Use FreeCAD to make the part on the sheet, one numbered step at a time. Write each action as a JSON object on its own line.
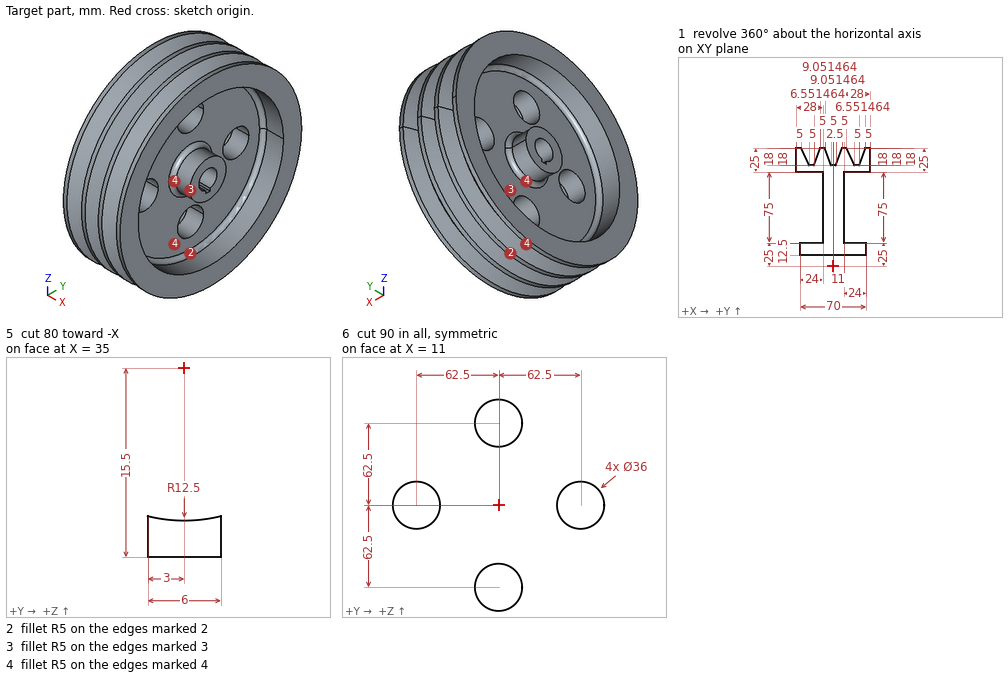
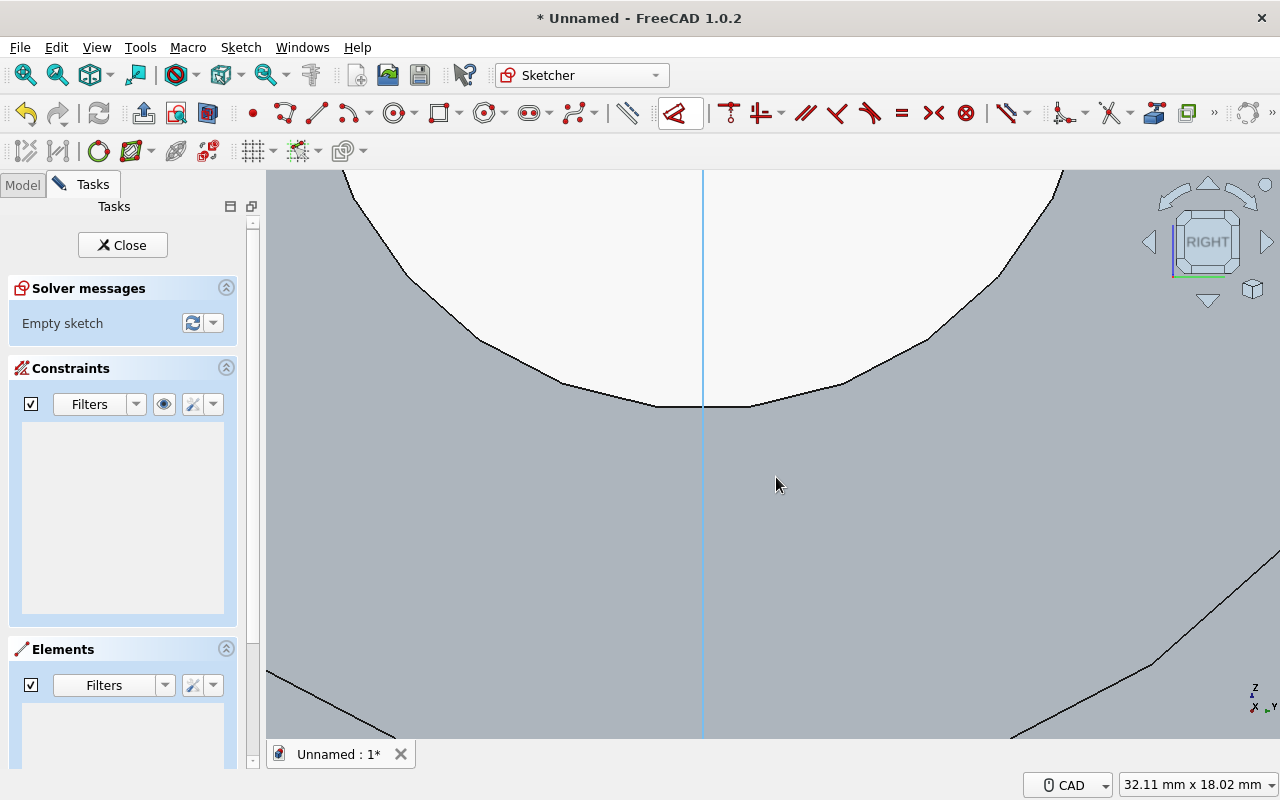
{"action": "scroll", "coordinate": [703, 450], "scroll_direction": "up", "scroll_amount": 6}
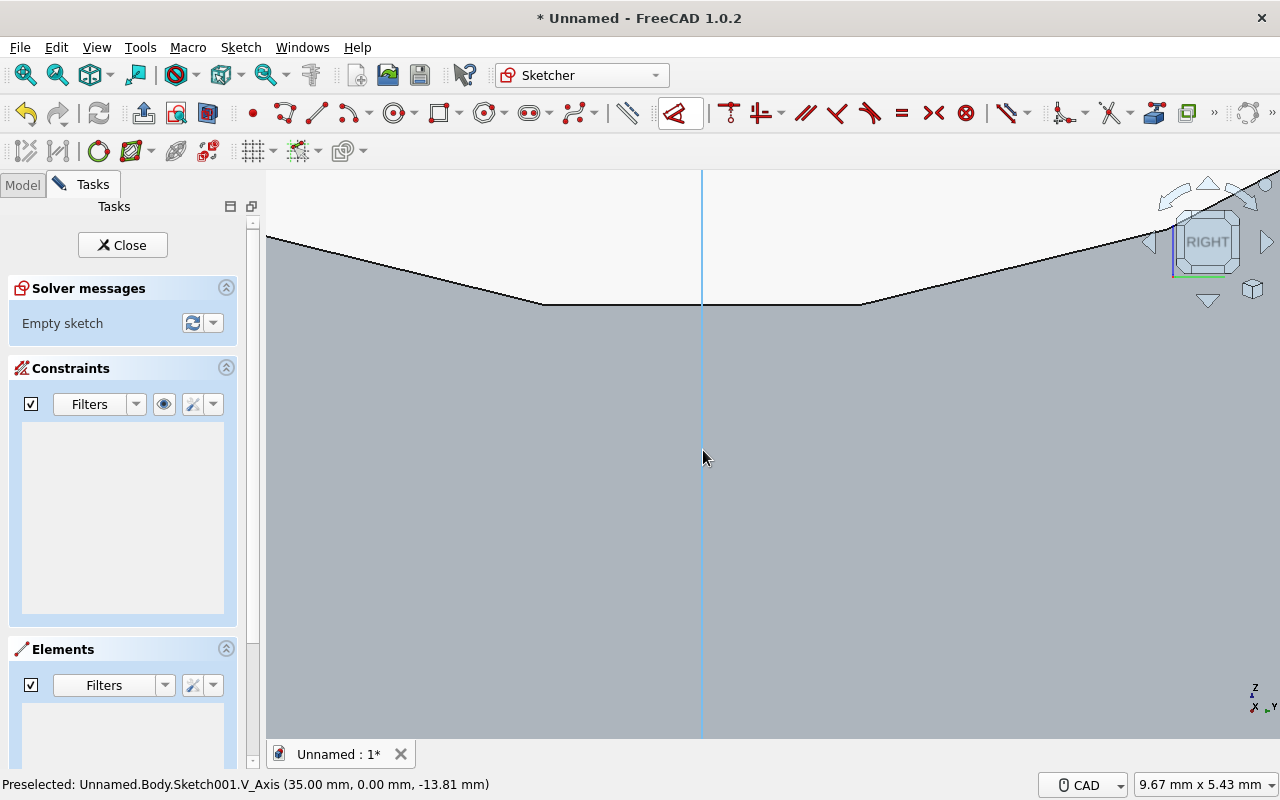
{"action": "left_click", "coordinate": [286, 114]}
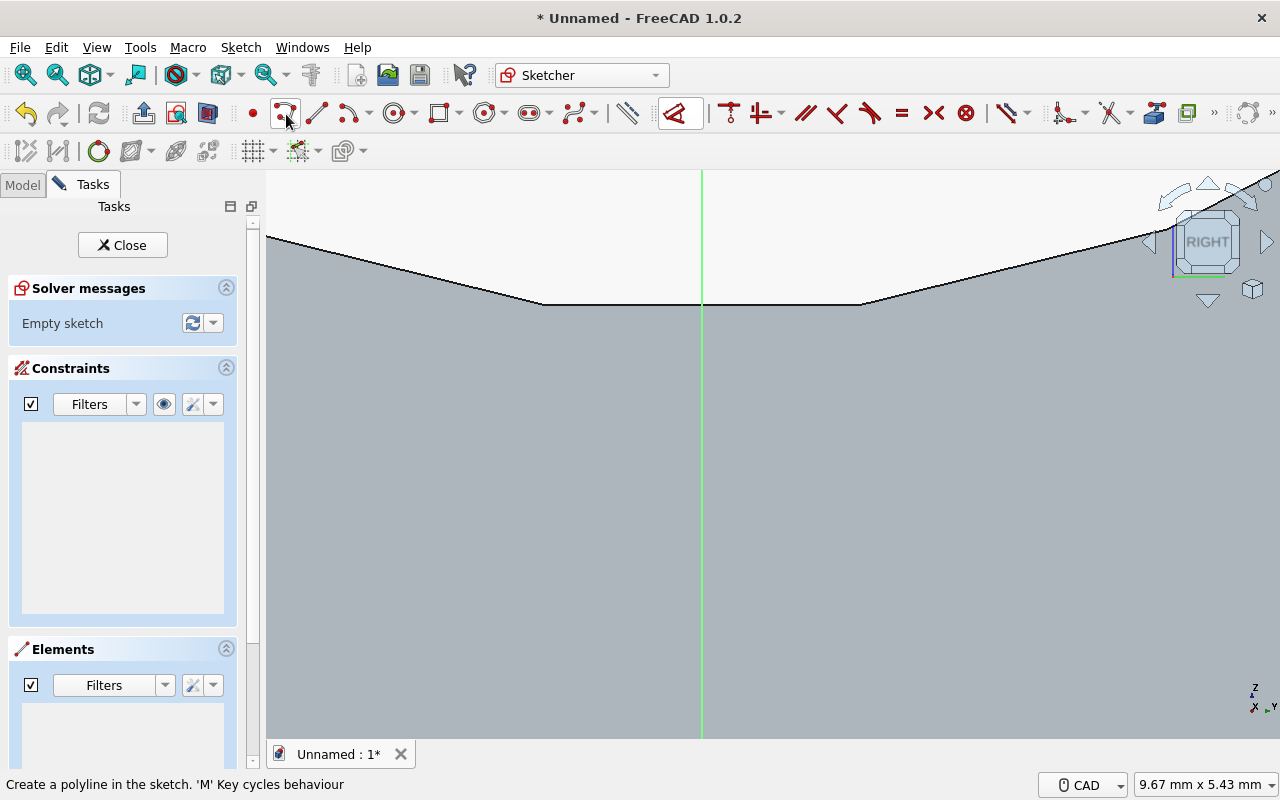
{"action": "left_click", "coordinate": [388, 276]}
{"action": "left_click", "coordinate": [388, 629]}
{"action": "left_click", "coordinate": [1017, 629]}
{"action": "left_click", "coordinate": [1017, 276]}
{"action": "right_click", "coordinate": [1017, 276]}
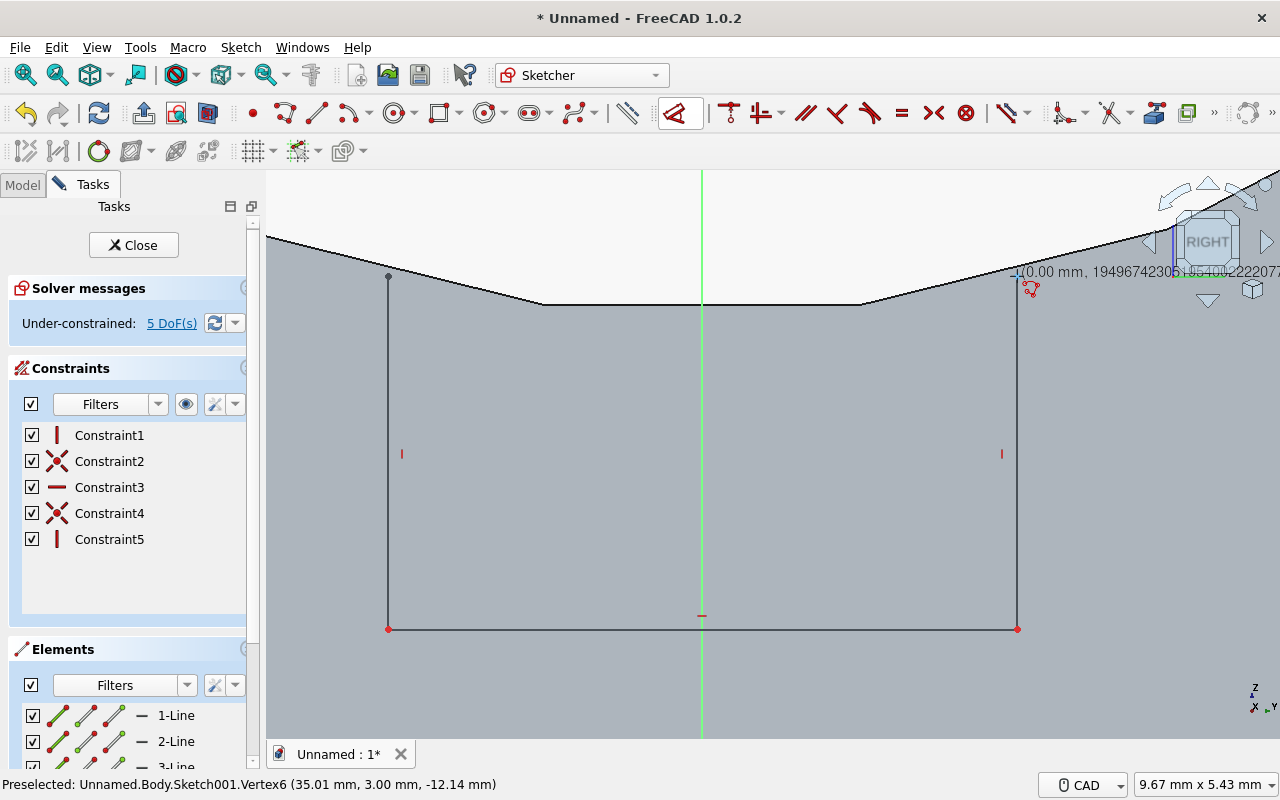
{"action": "left_click", "coordinate": [372, 114]}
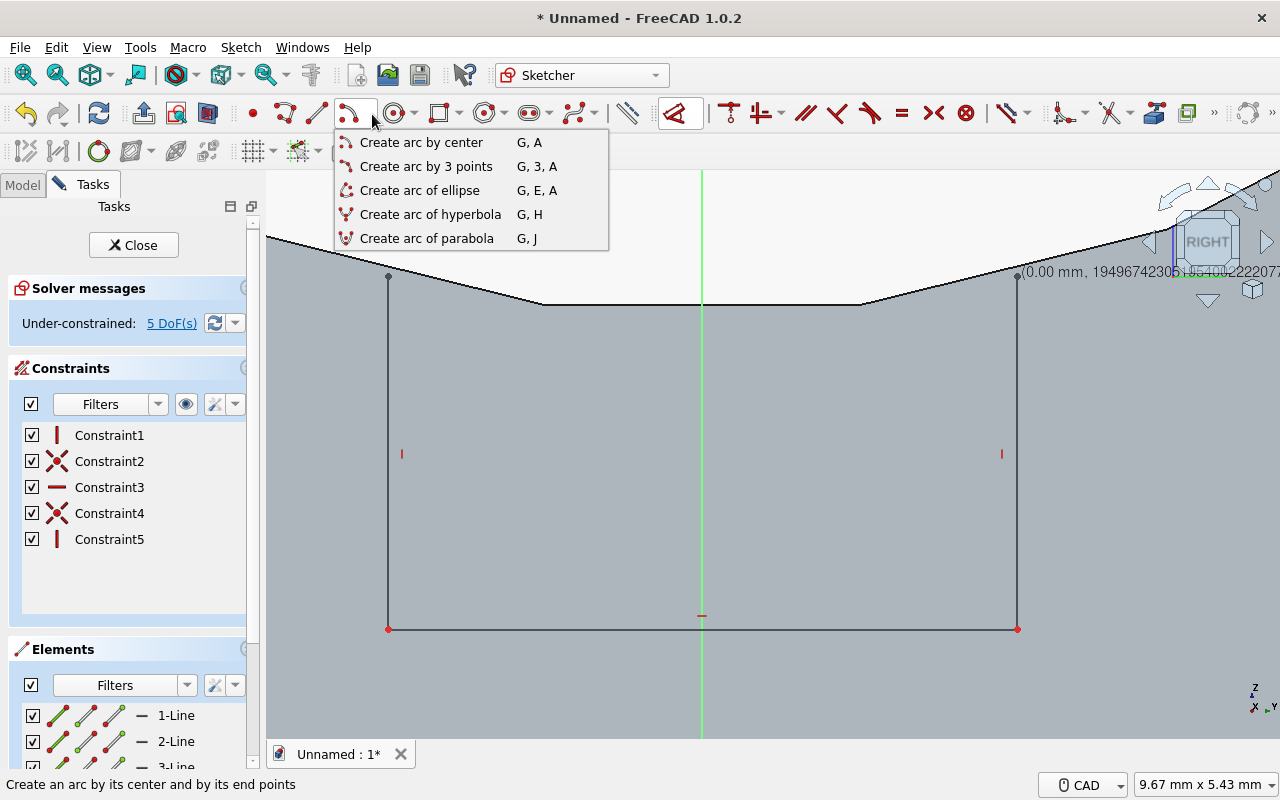
{"action": "left_click", "coordinate": [472, 166]}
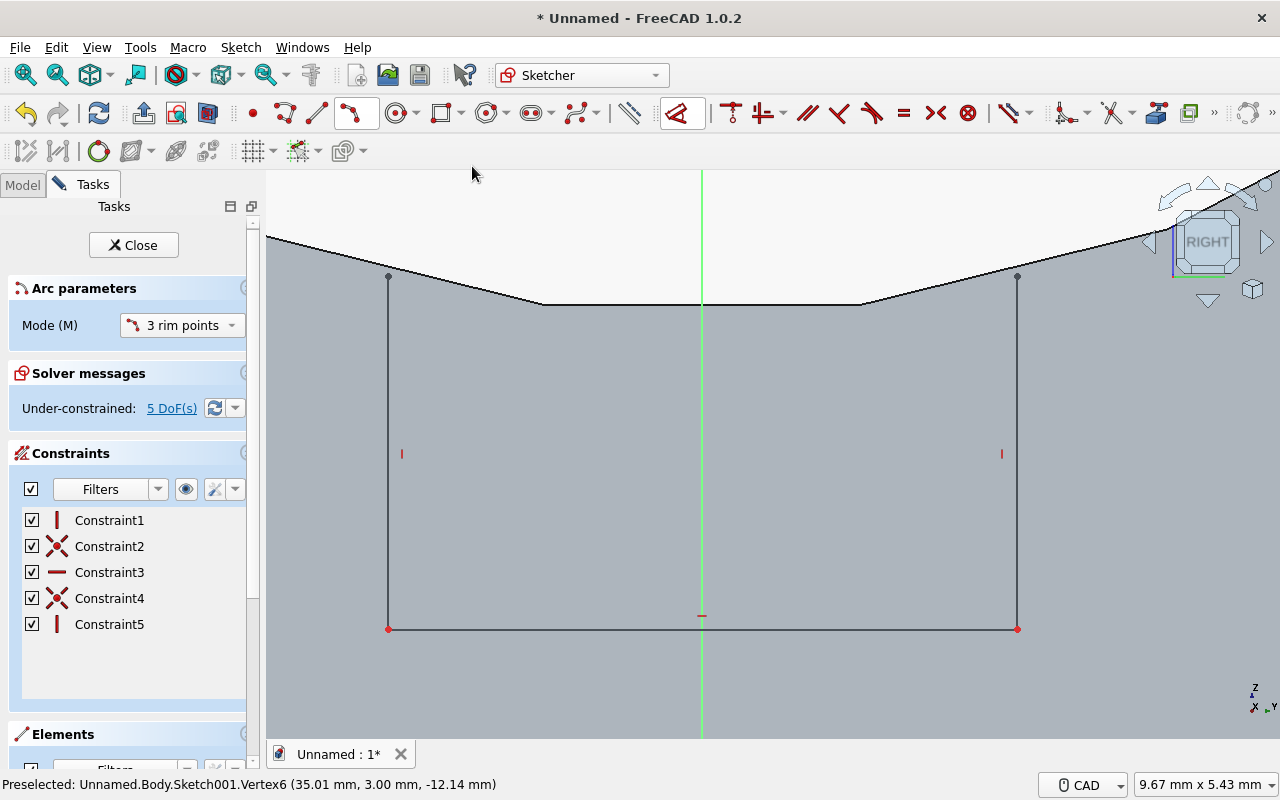
{"action": "left_click", "coordinate": [1017, 277]}
{"action": "left_click", "coordinate": [388, 277]}
{"action": "left_click", "coordinate": [639, 313]}
{"action": "key", "text": "Escape"}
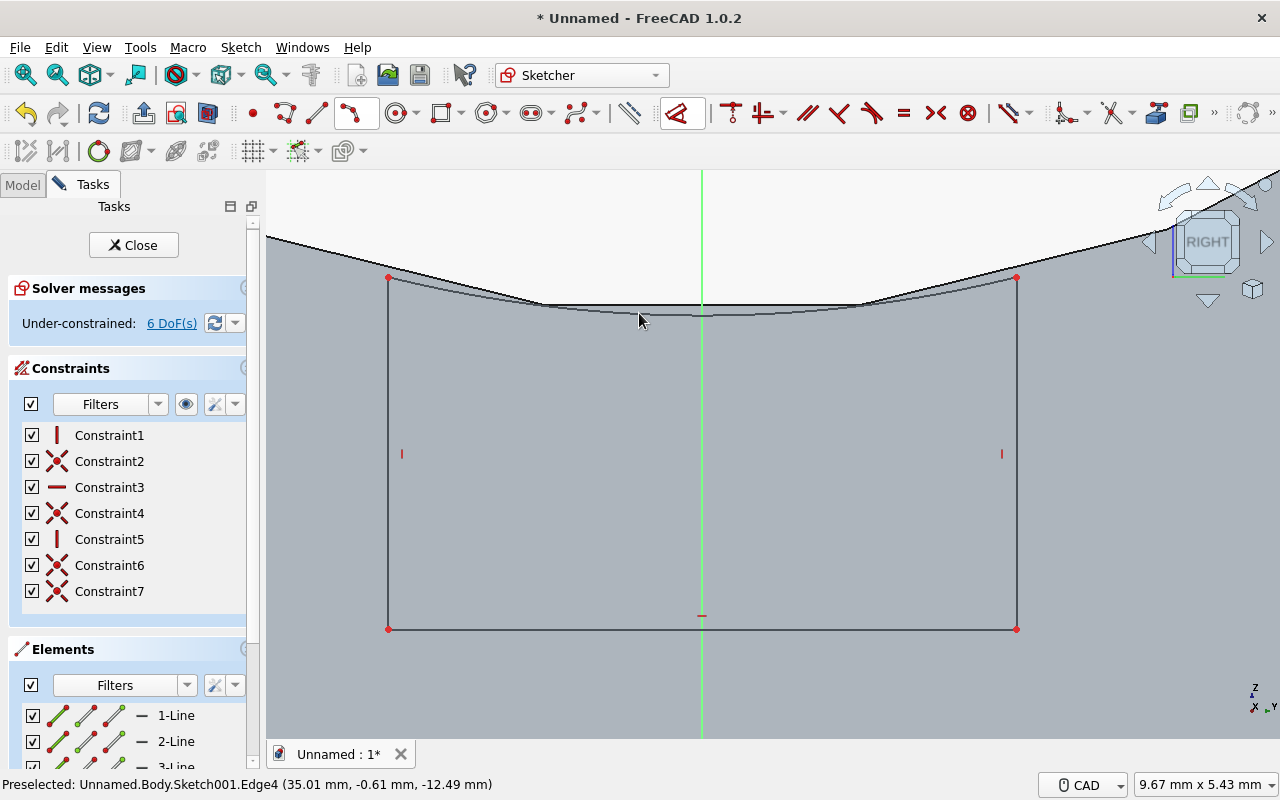
{"action": "scroll", "coordinate": [705, 663], "scroll_direction": "down", "scroll_amount": 7}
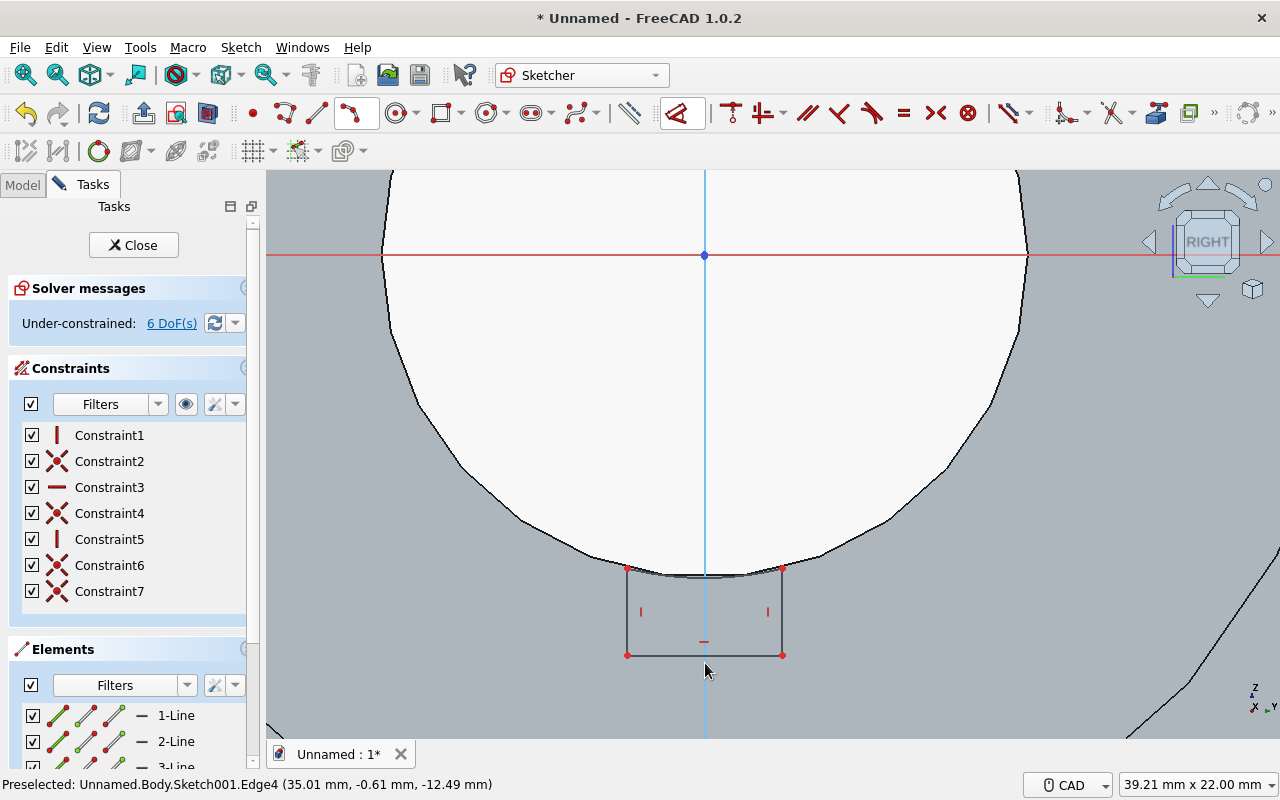
{"action": "left_click_drag", "start_coordinate": [695, 245], "coordinate": [715, 267]}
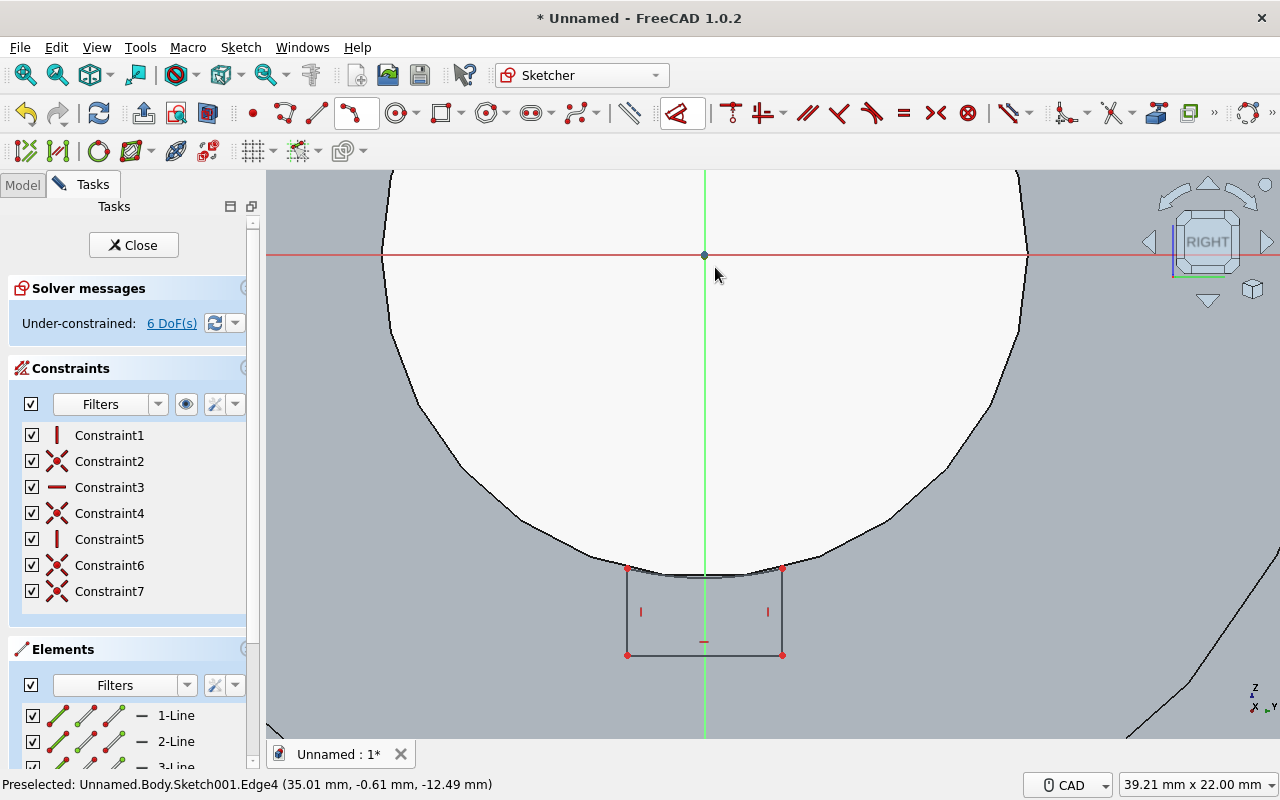
{"action": "left_click", "coordinate": [732, 114]}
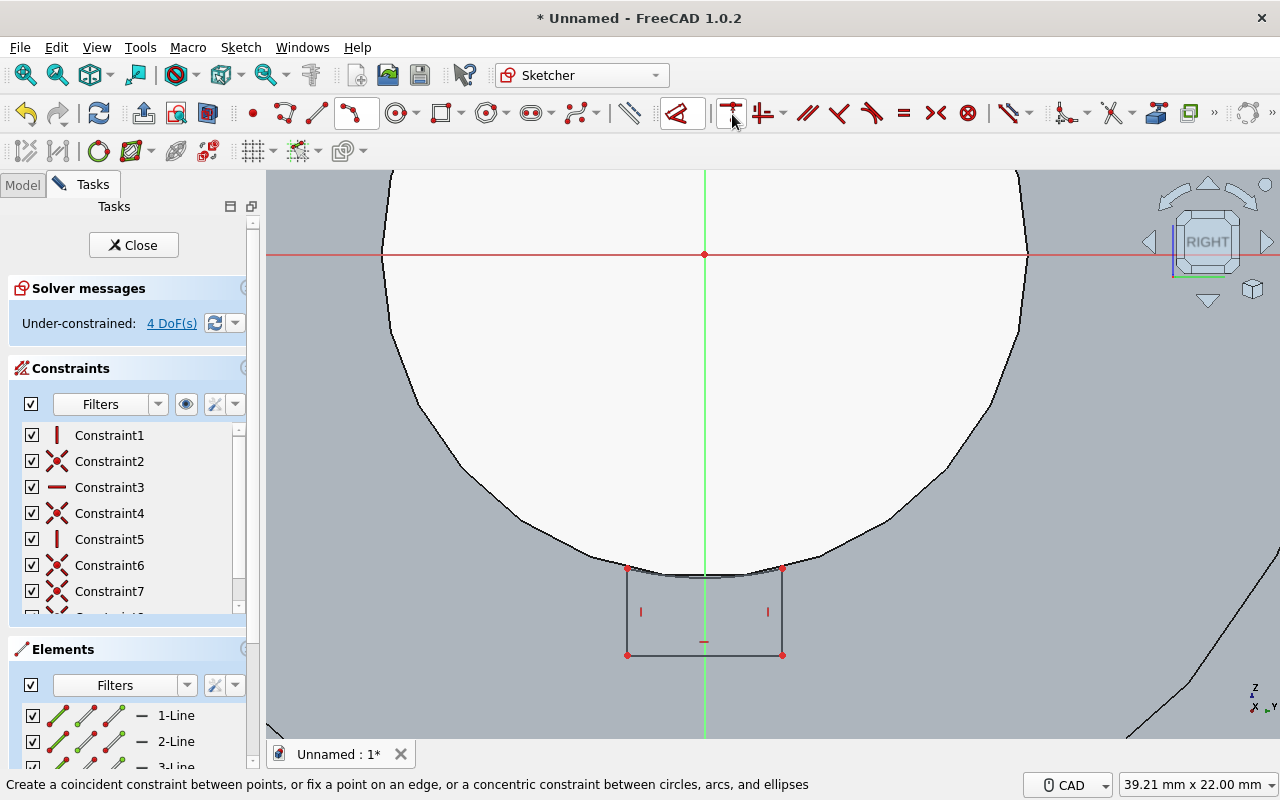
{"action": "left_click", "coordinate": [673, 576]}